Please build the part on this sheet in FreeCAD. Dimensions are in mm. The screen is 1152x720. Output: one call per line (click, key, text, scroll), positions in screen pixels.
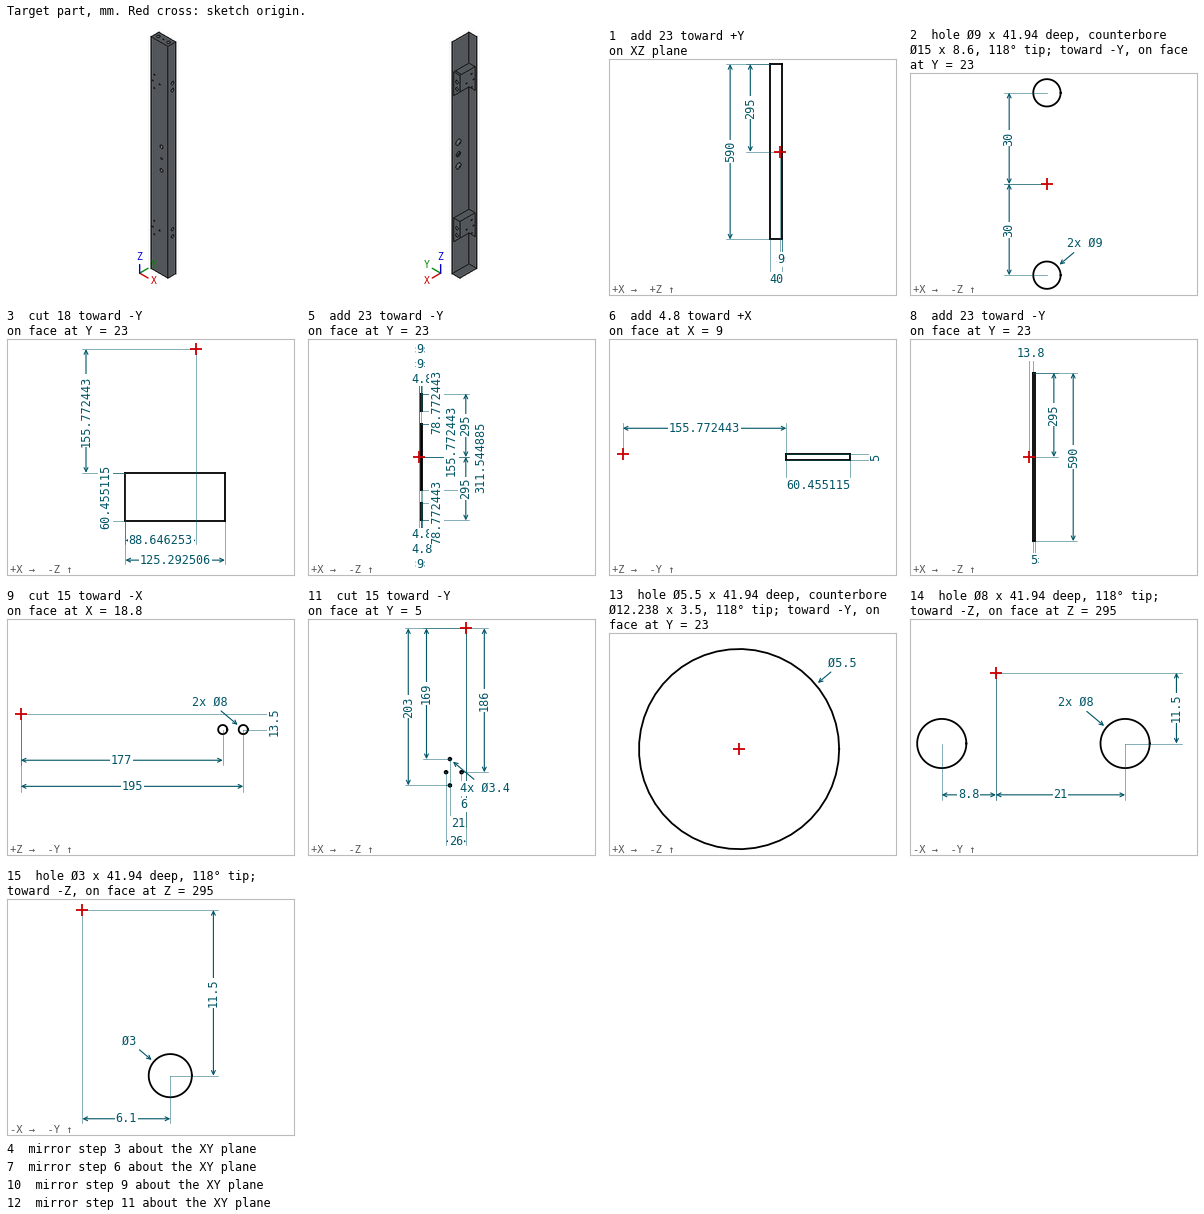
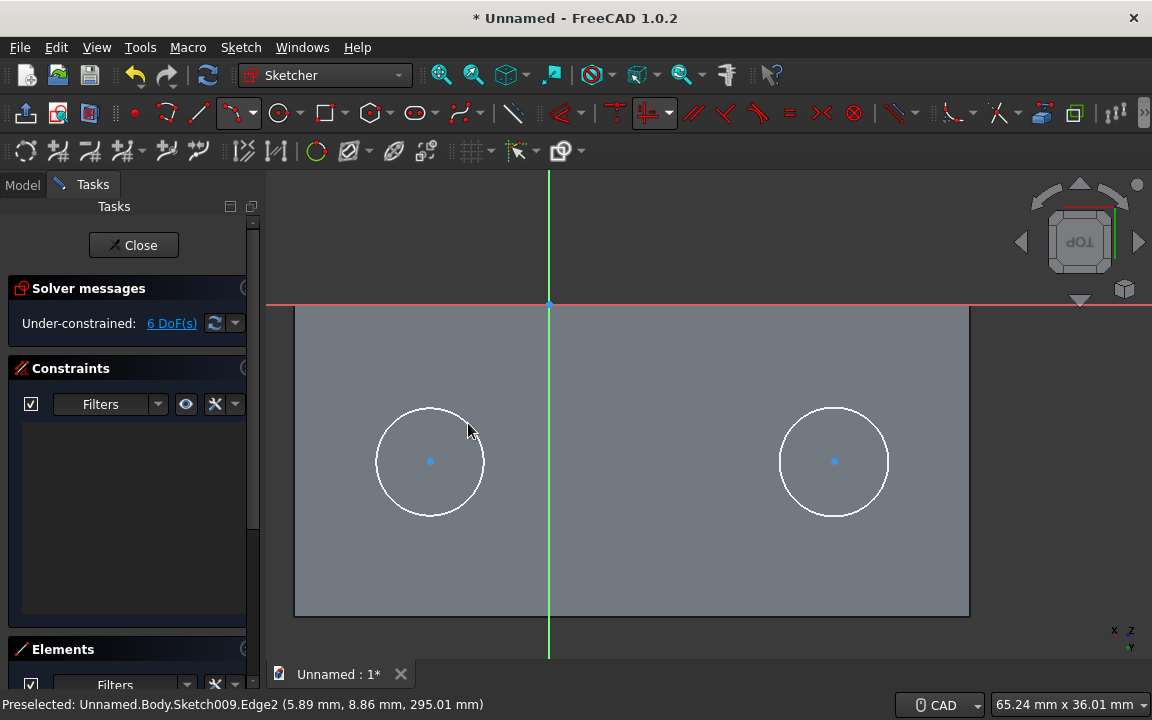
click(872, 423)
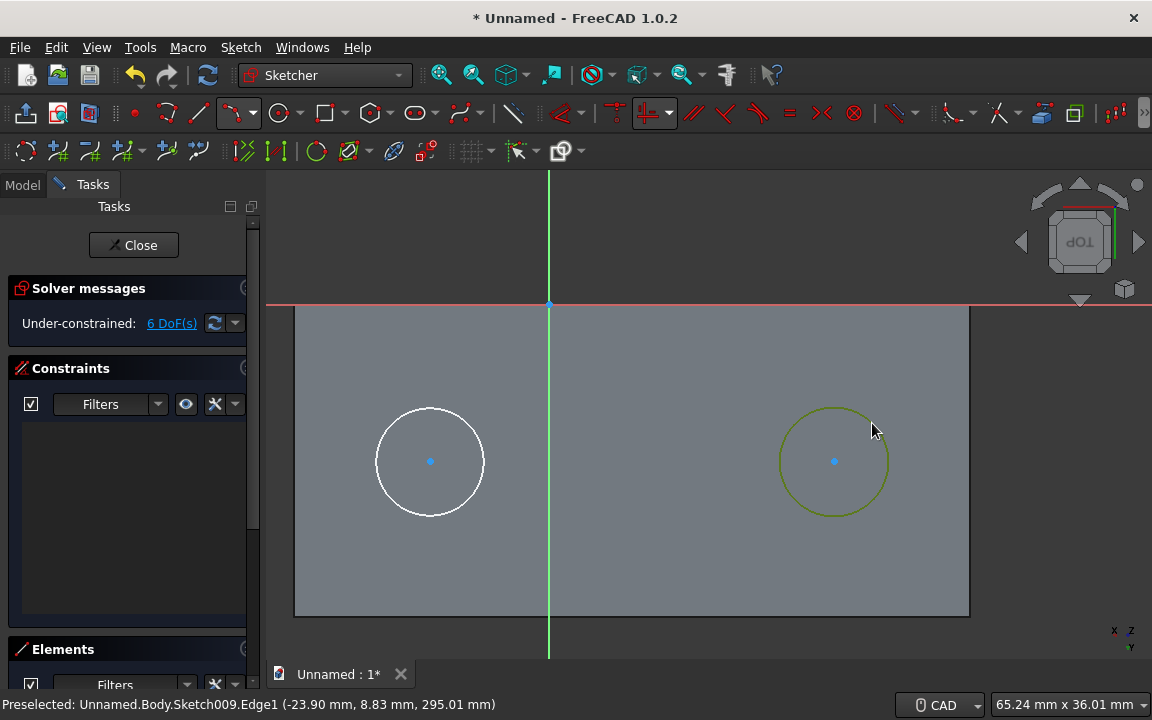
click(468, 424)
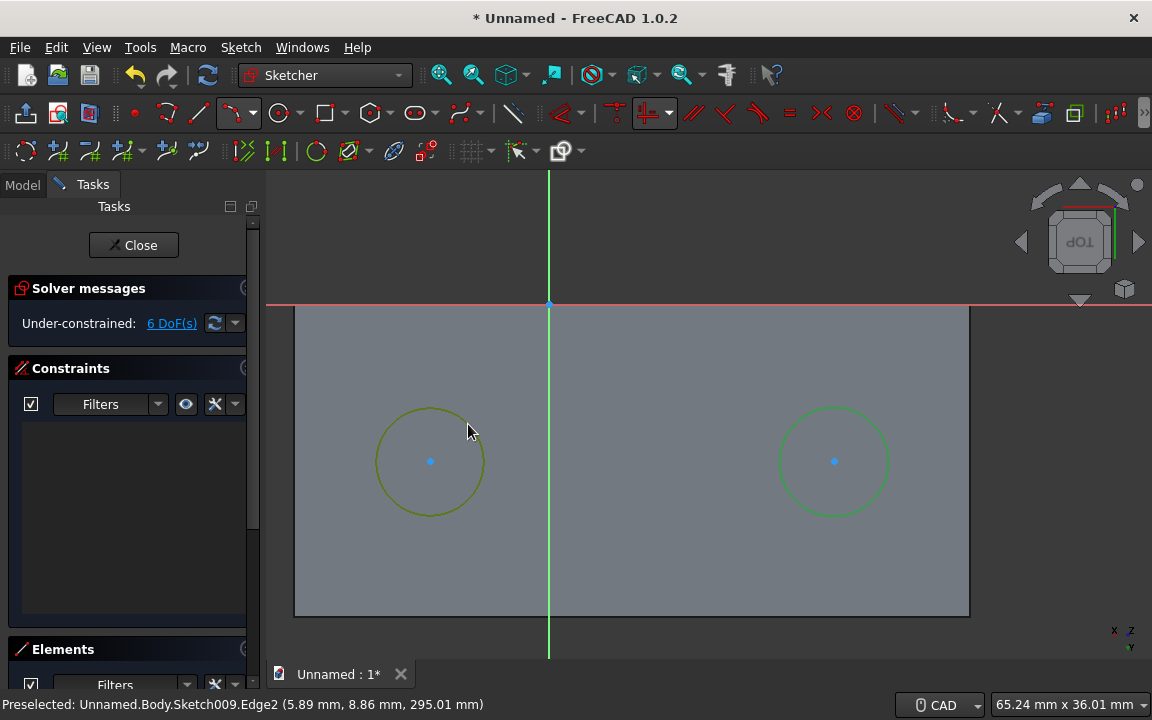
click(790, 114)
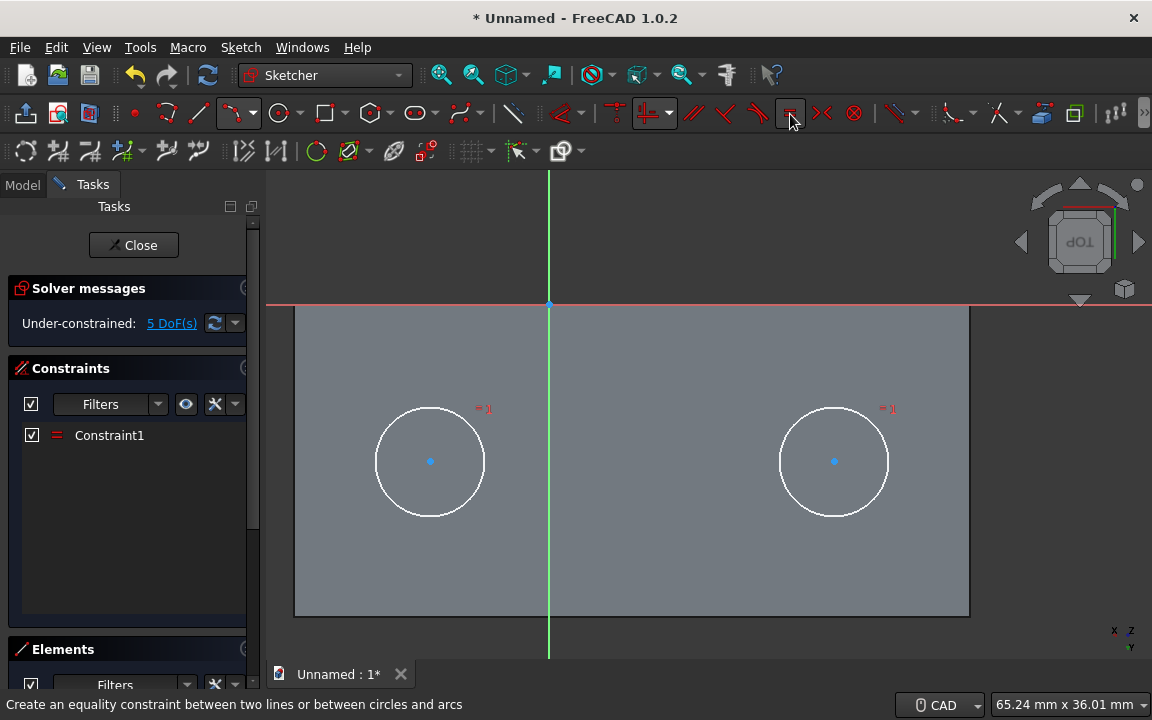
click(834, 462)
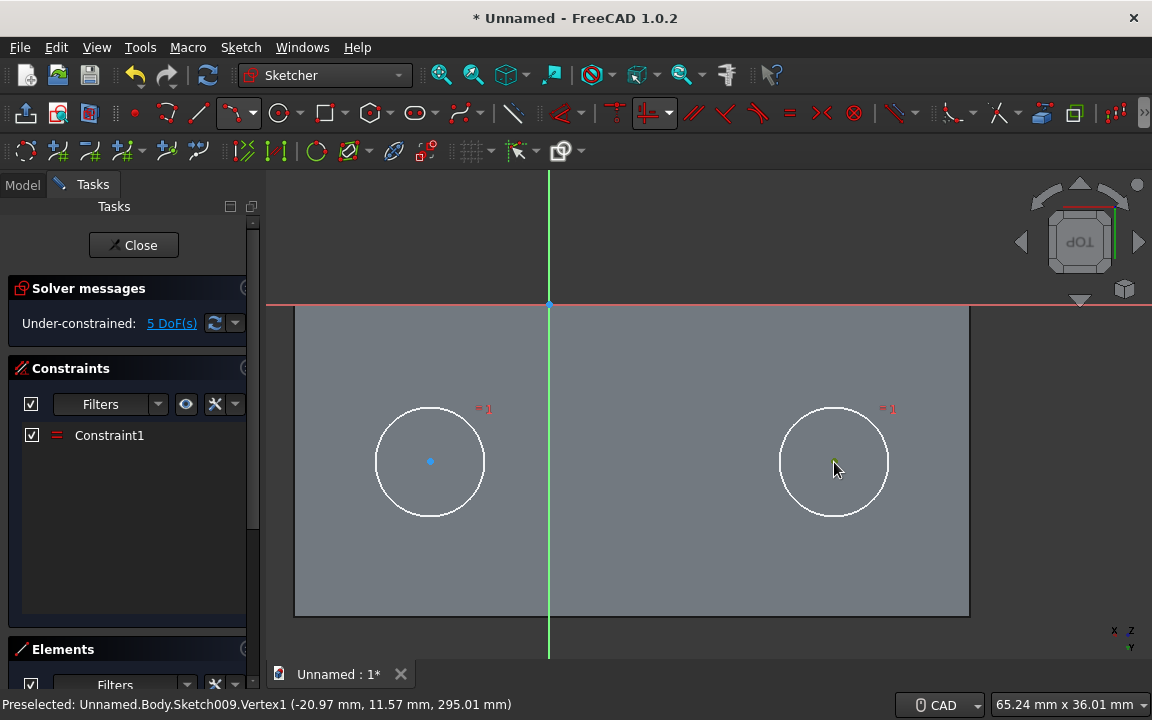
click(430, 462)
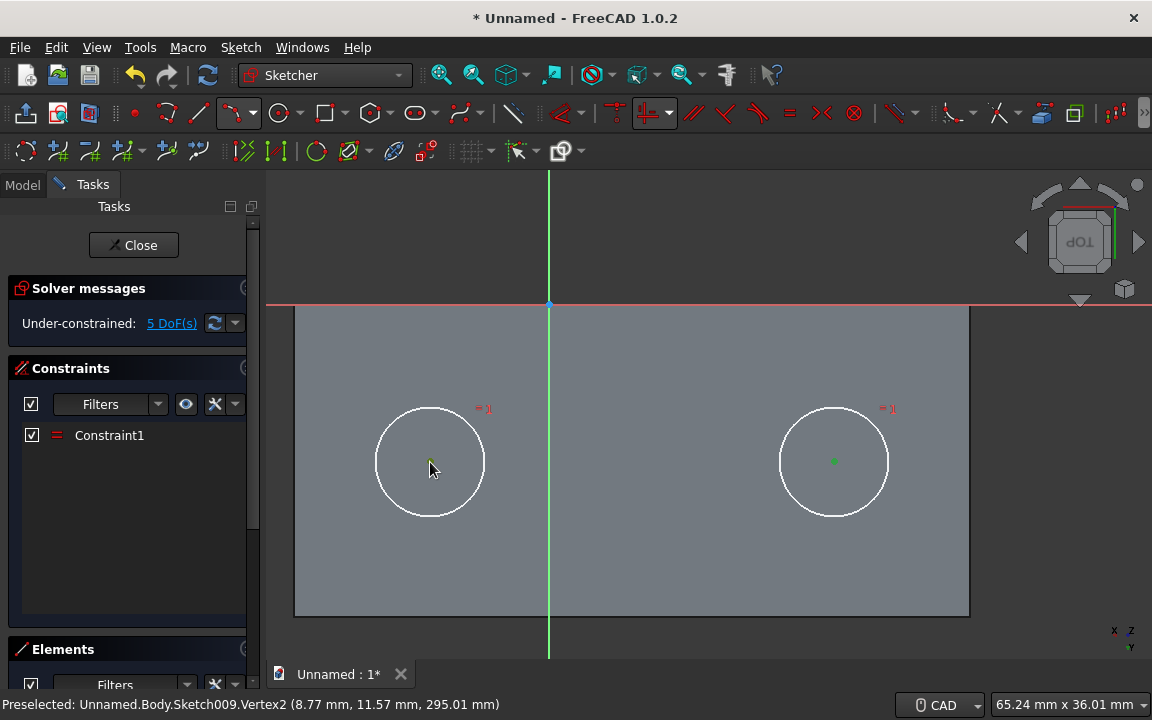
key(h)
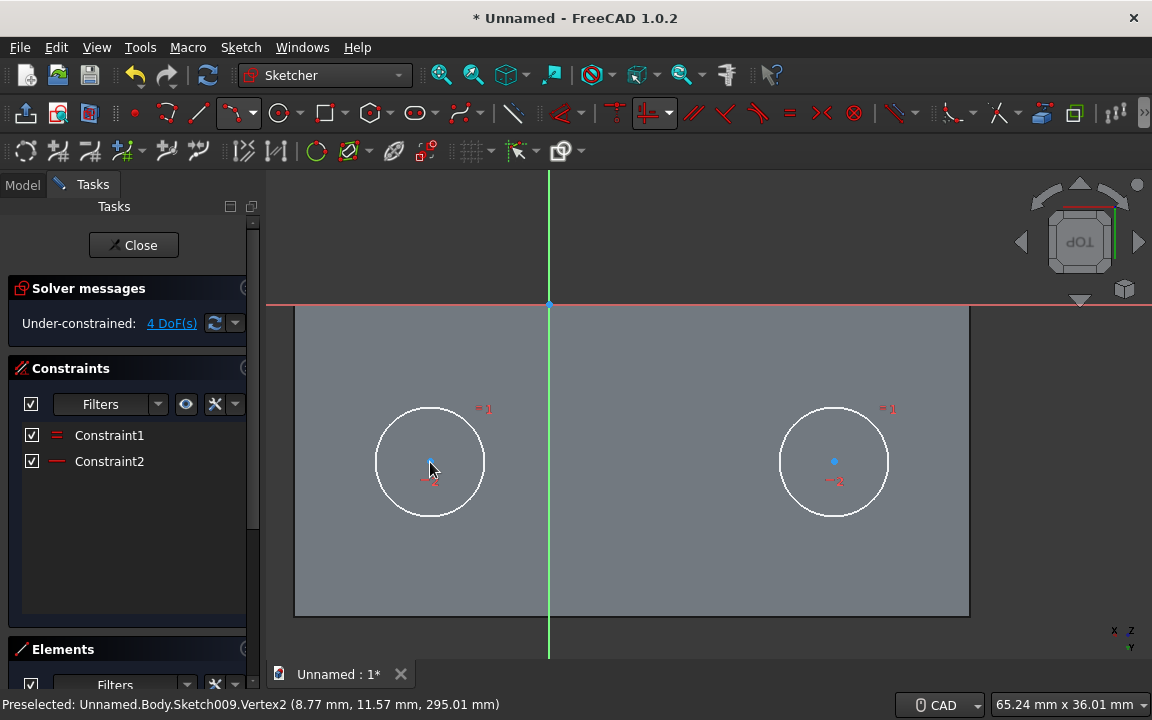
click(560, 114)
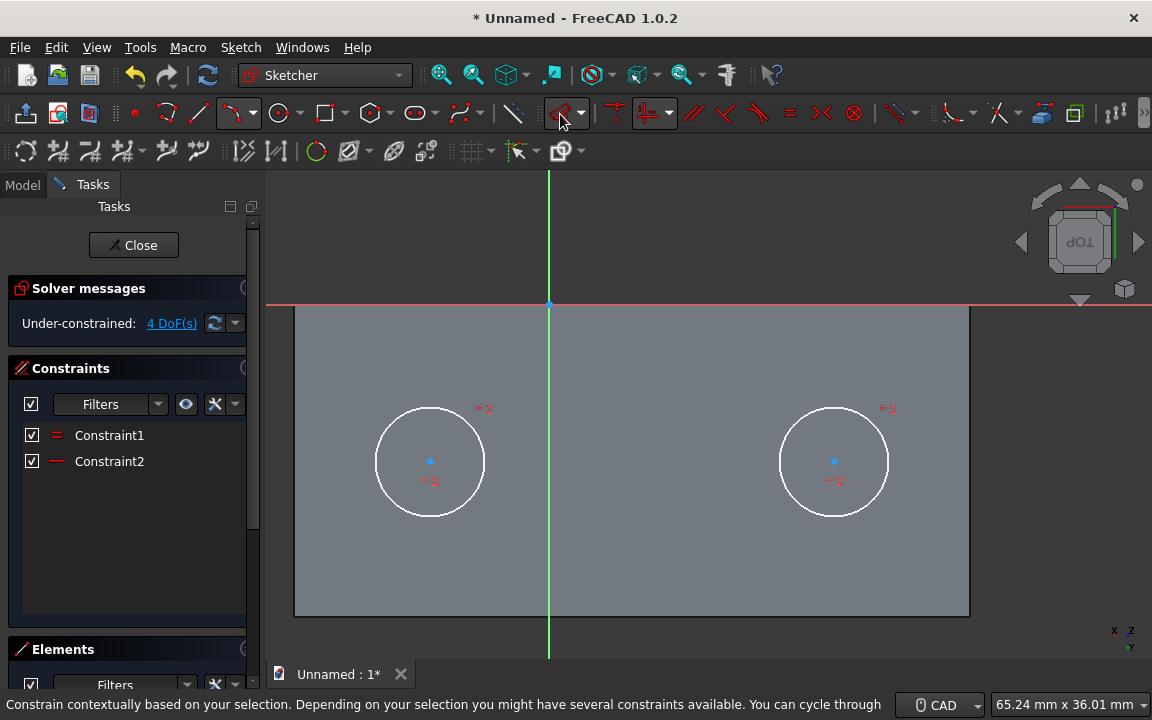
click(872, 423)
click(894, 400)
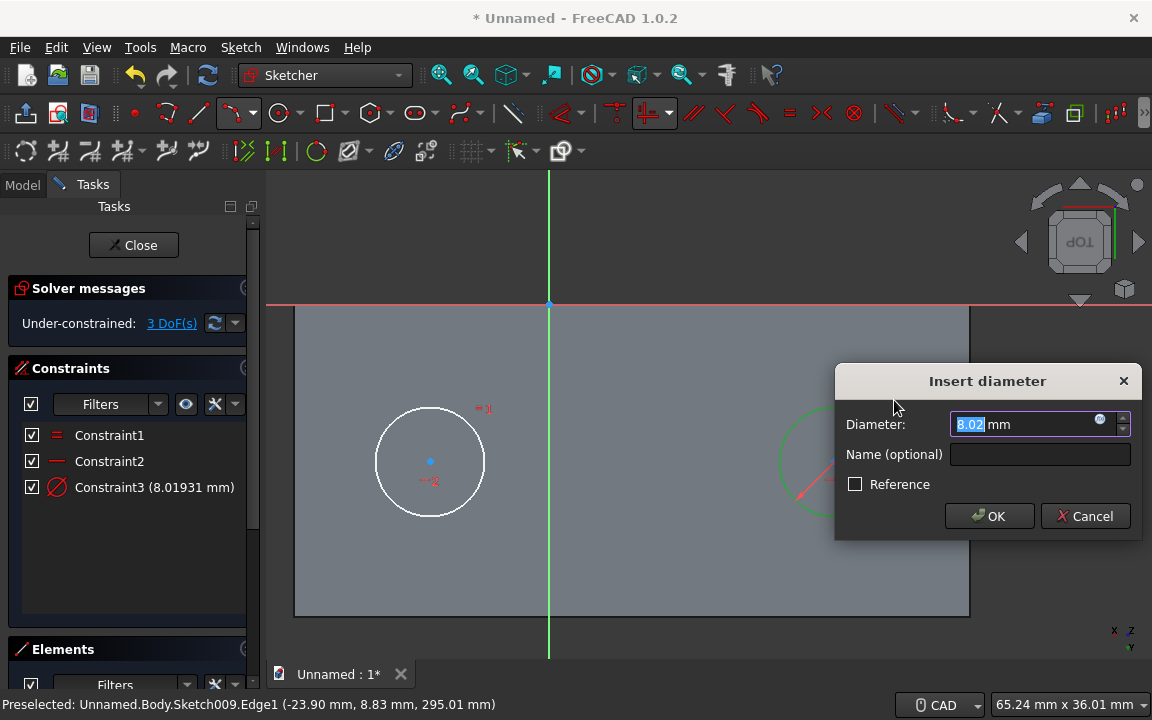
text(8)
key(Return)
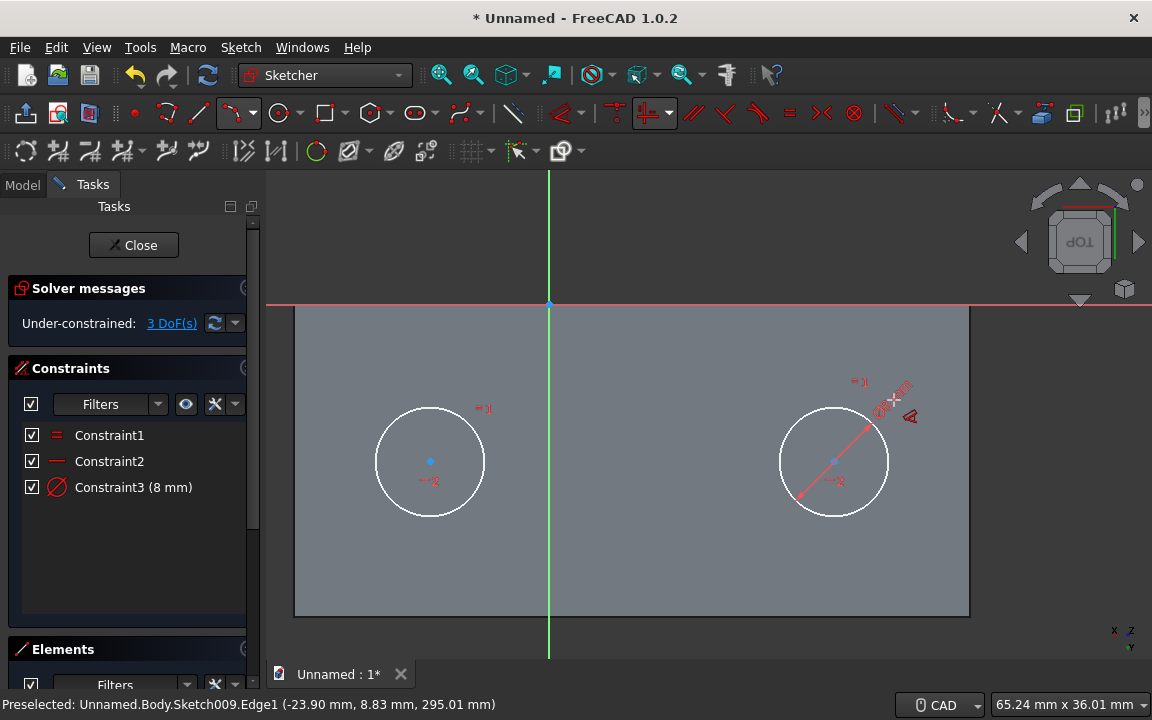
click(834, 462)
click(692, 271)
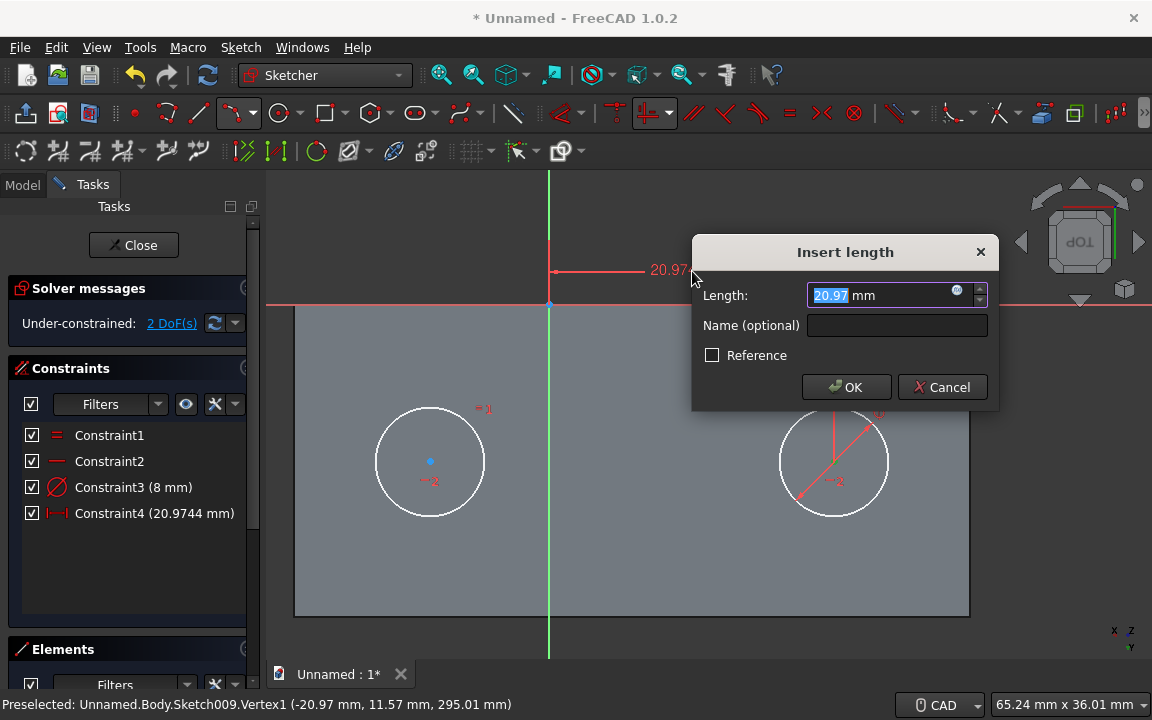
text(21)
key(Return)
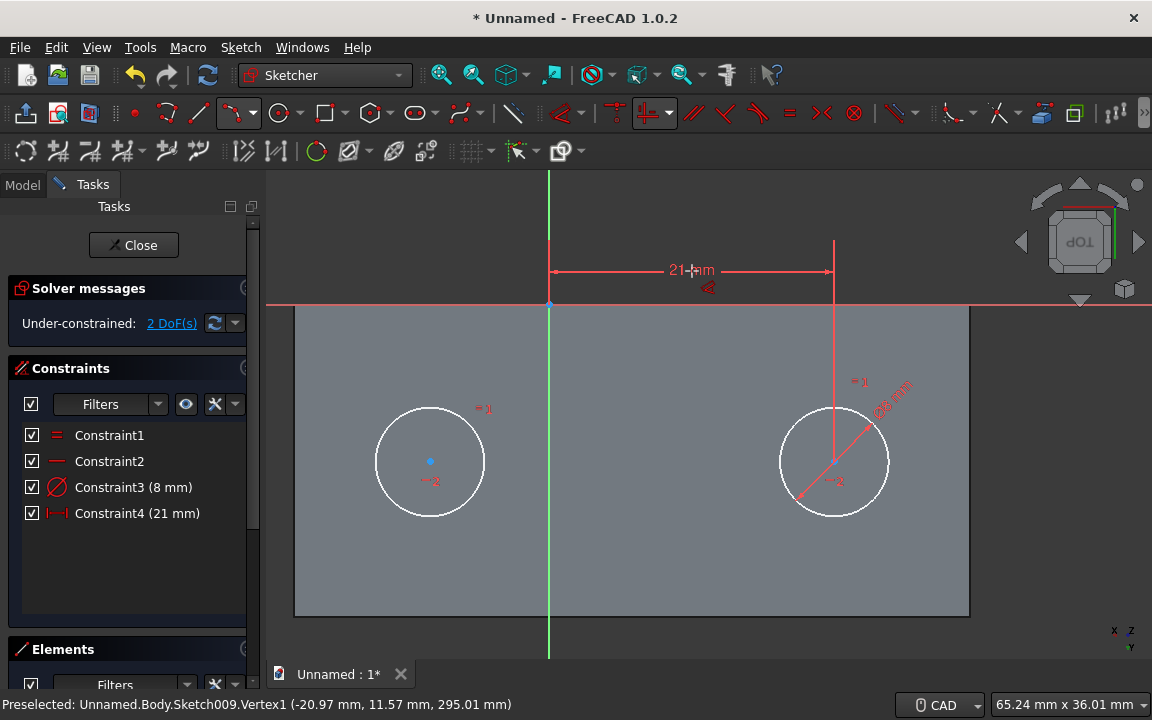
click(430, 462)
click(490, 271)